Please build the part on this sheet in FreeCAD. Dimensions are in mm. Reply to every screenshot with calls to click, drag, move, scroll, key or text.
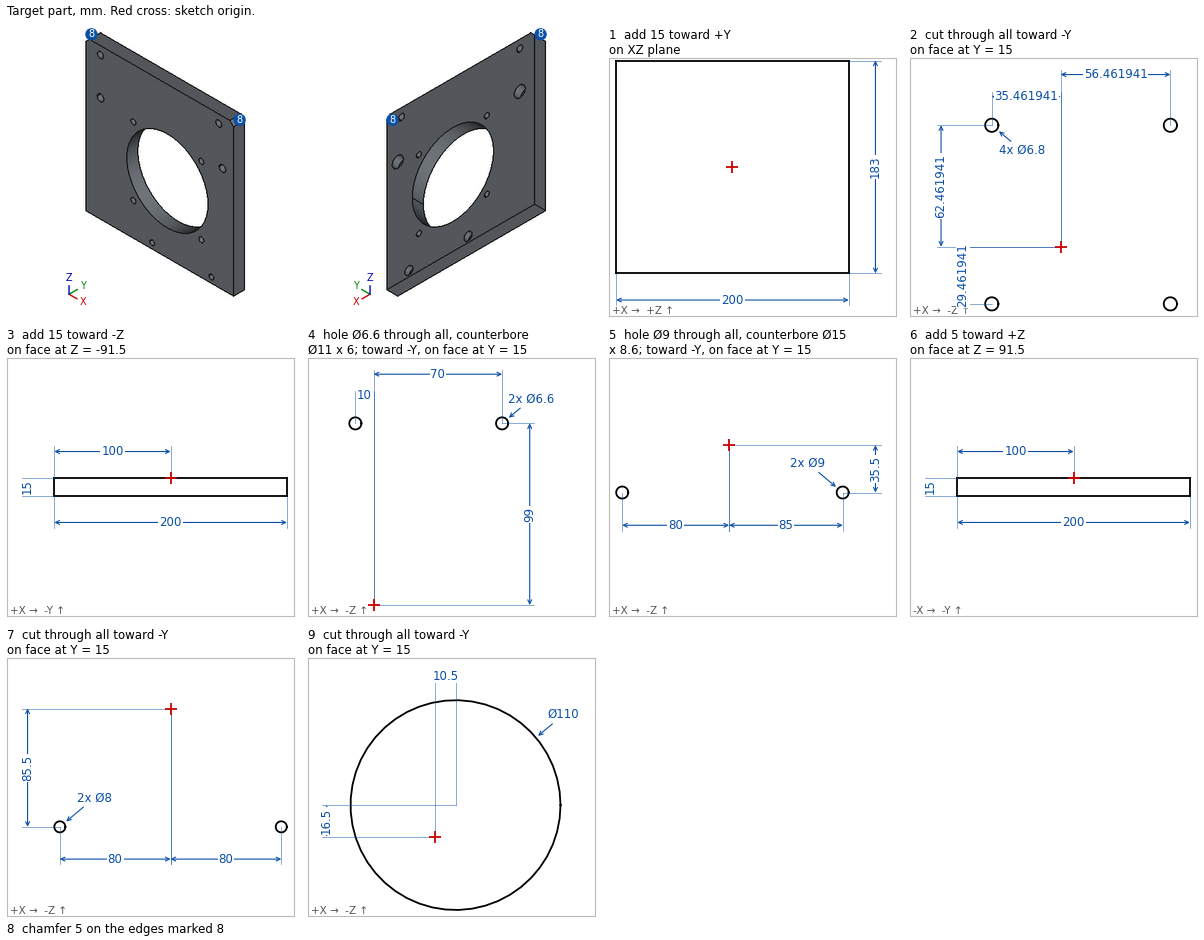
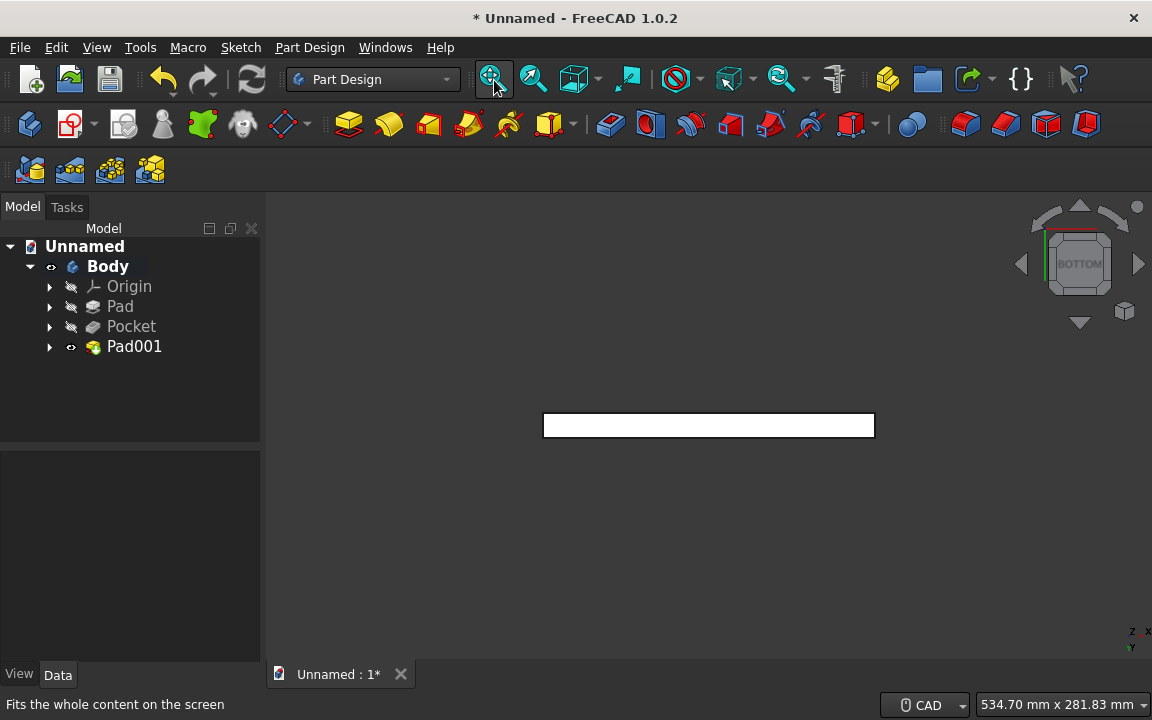
key(4)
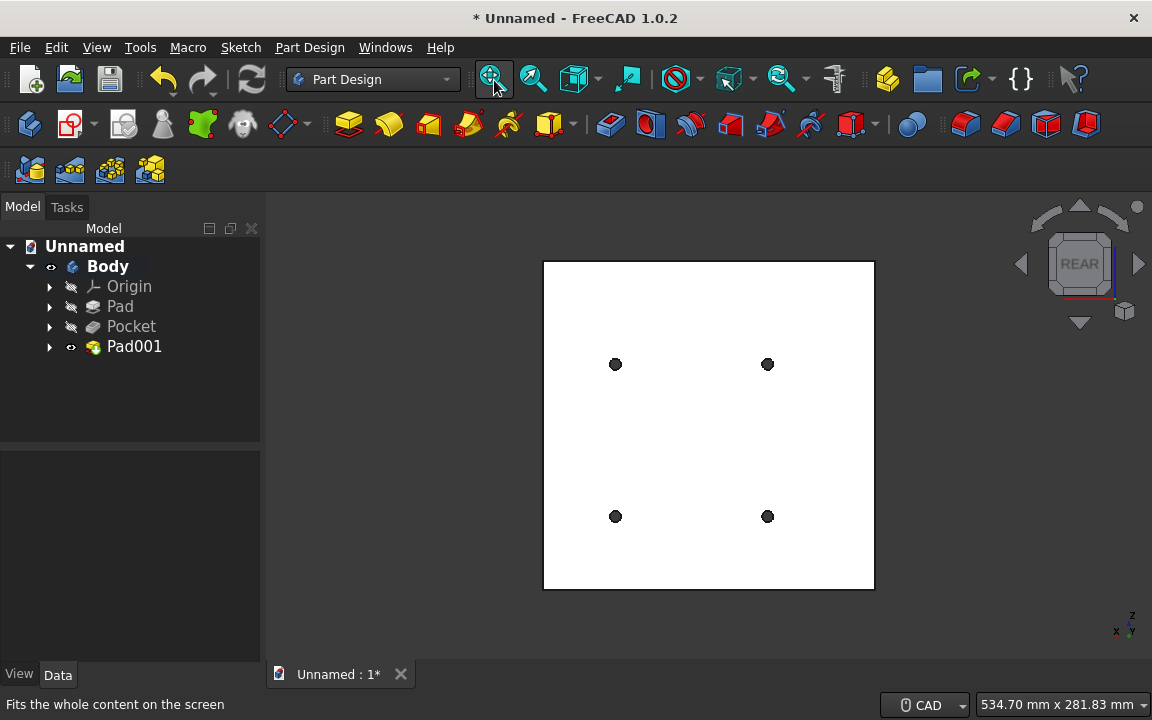
click(709, 424)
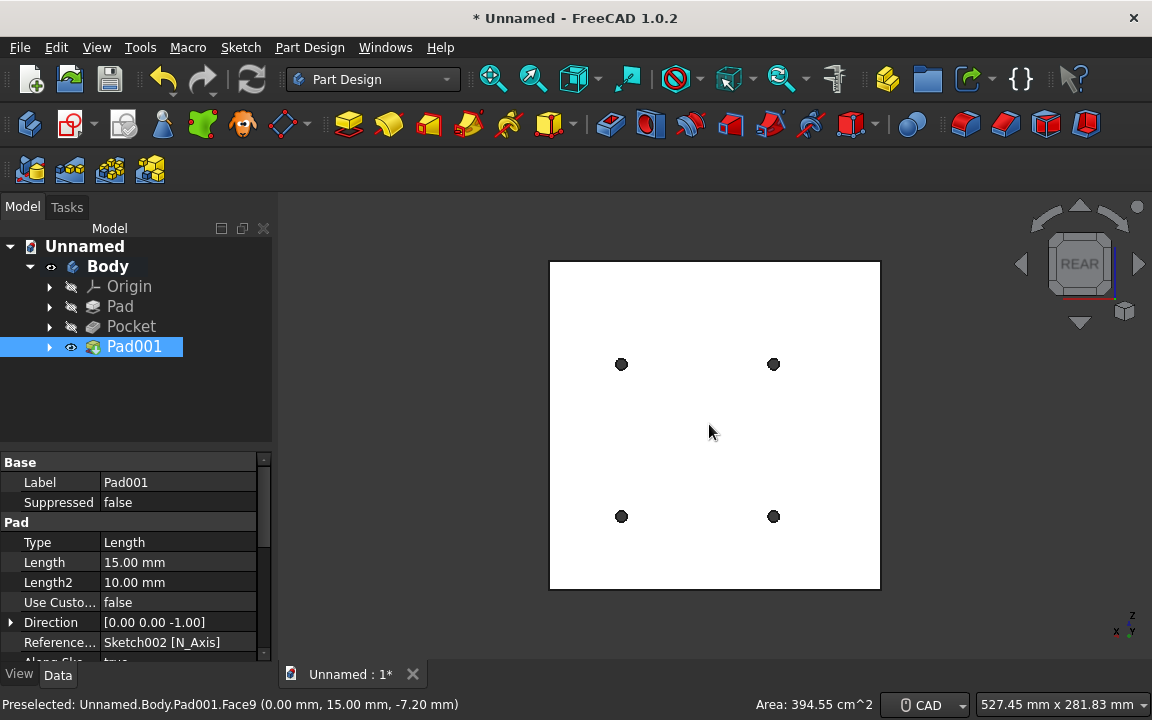
click(70, 124)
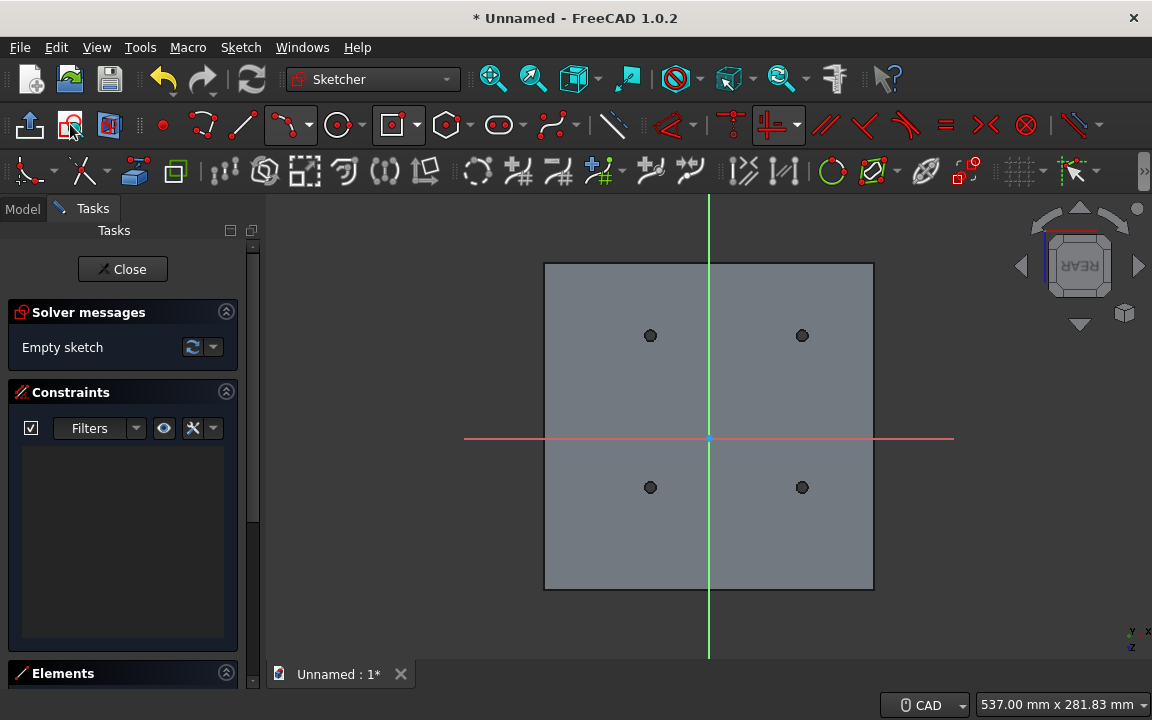
scroll(902, 267, up, 3)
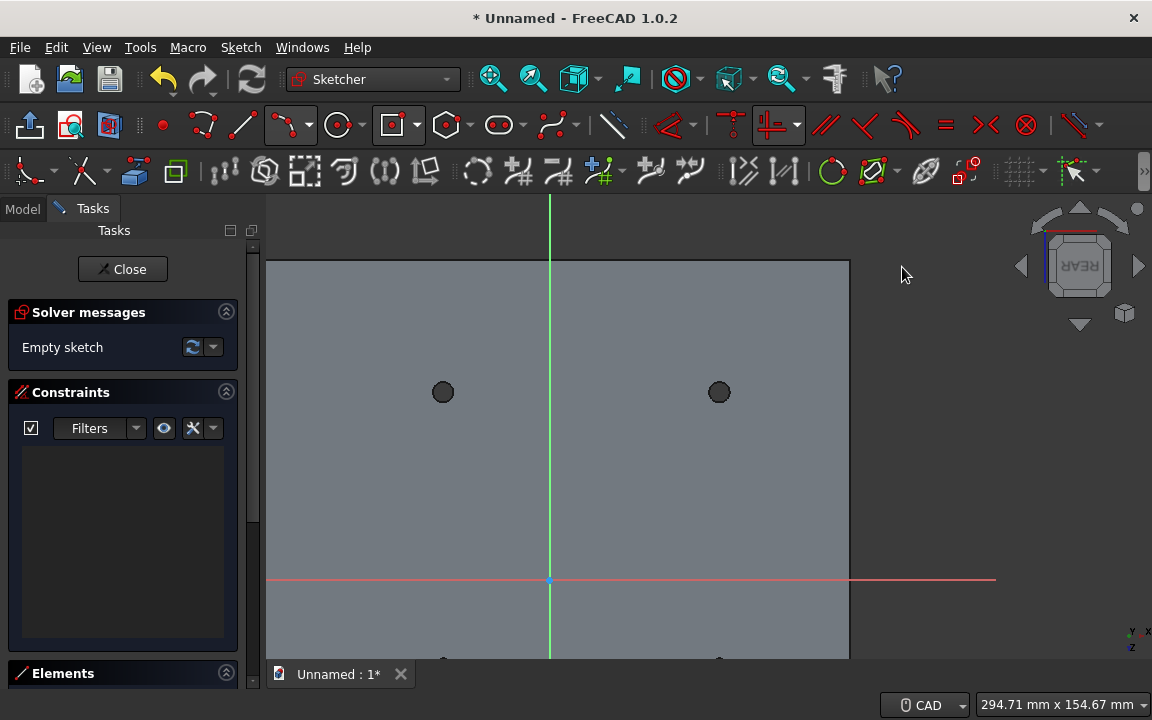
click(338, 126)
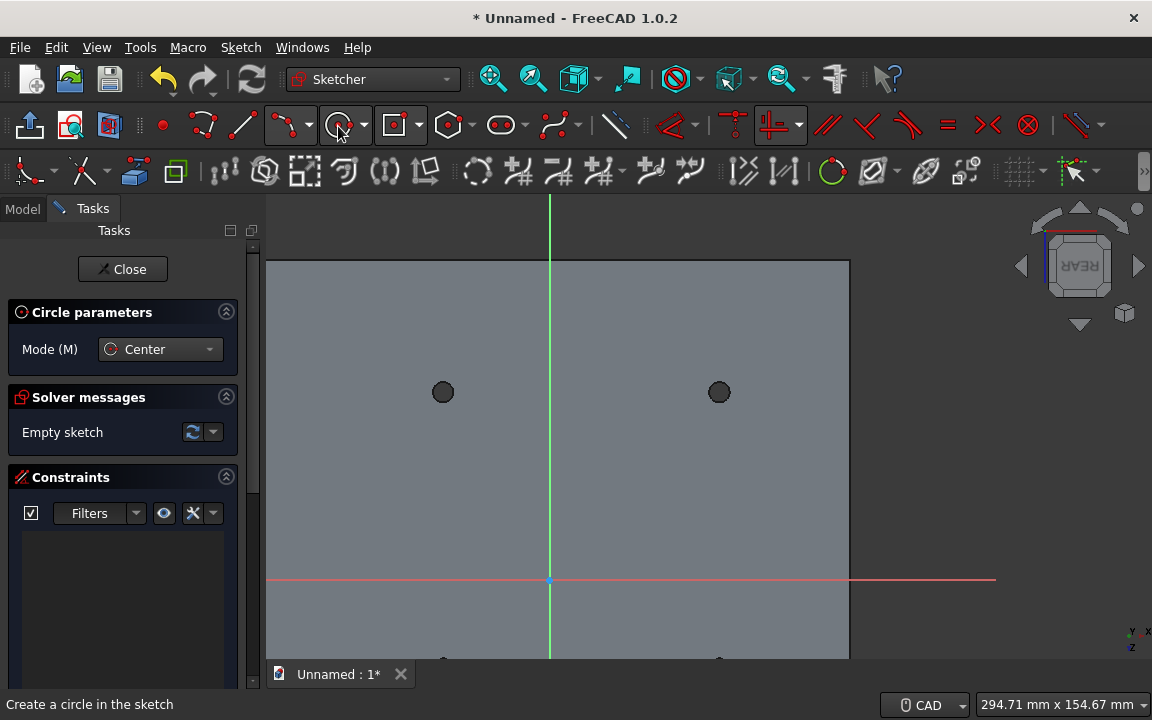
scroll(760, 282, up, 5)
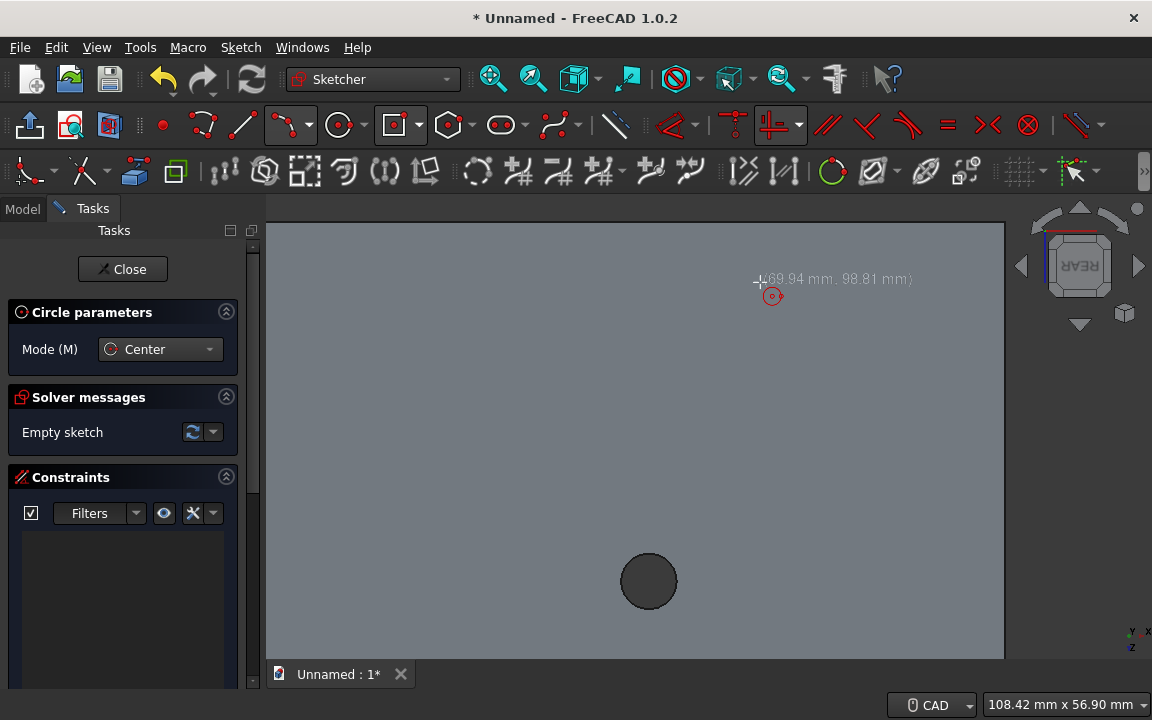
click(760, 283)
click(779, 264)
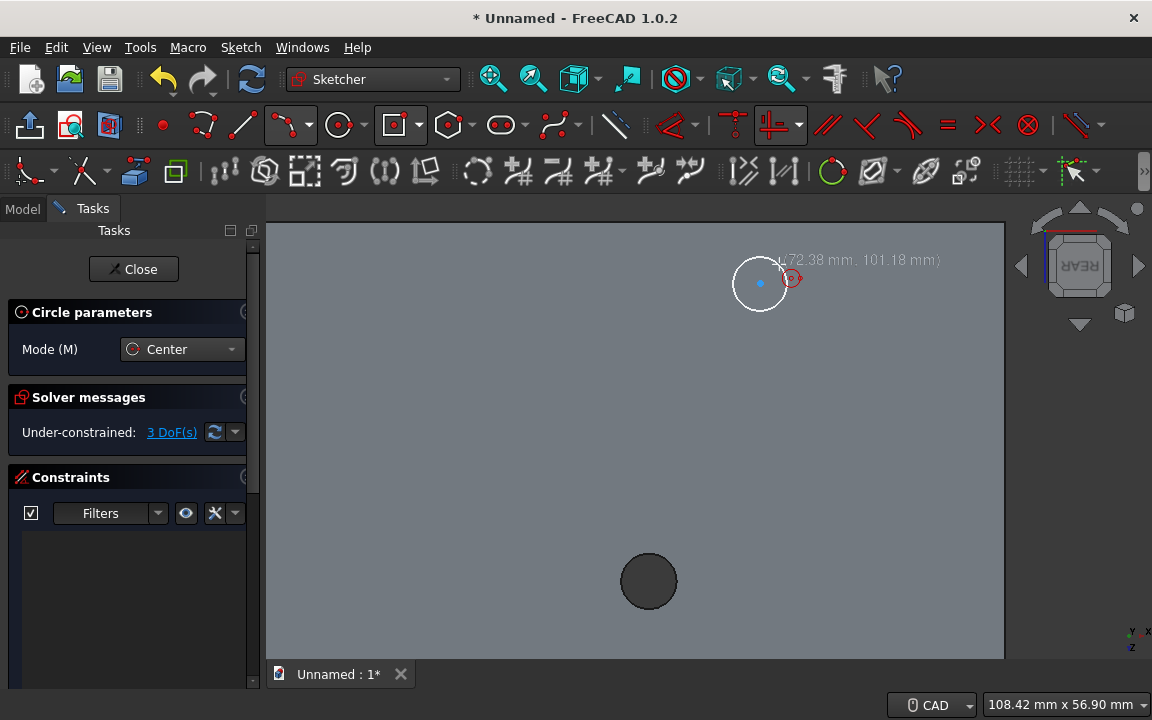
scroll(761, 283, down, 5)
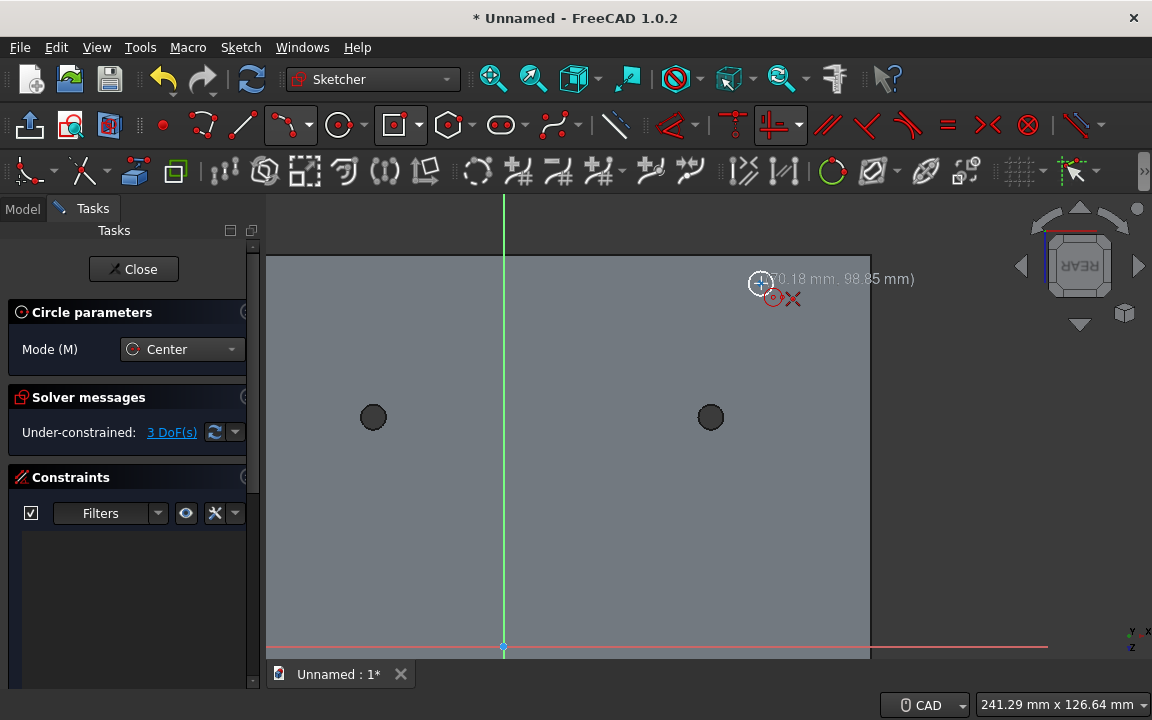
scroll(520, 283, up, 5)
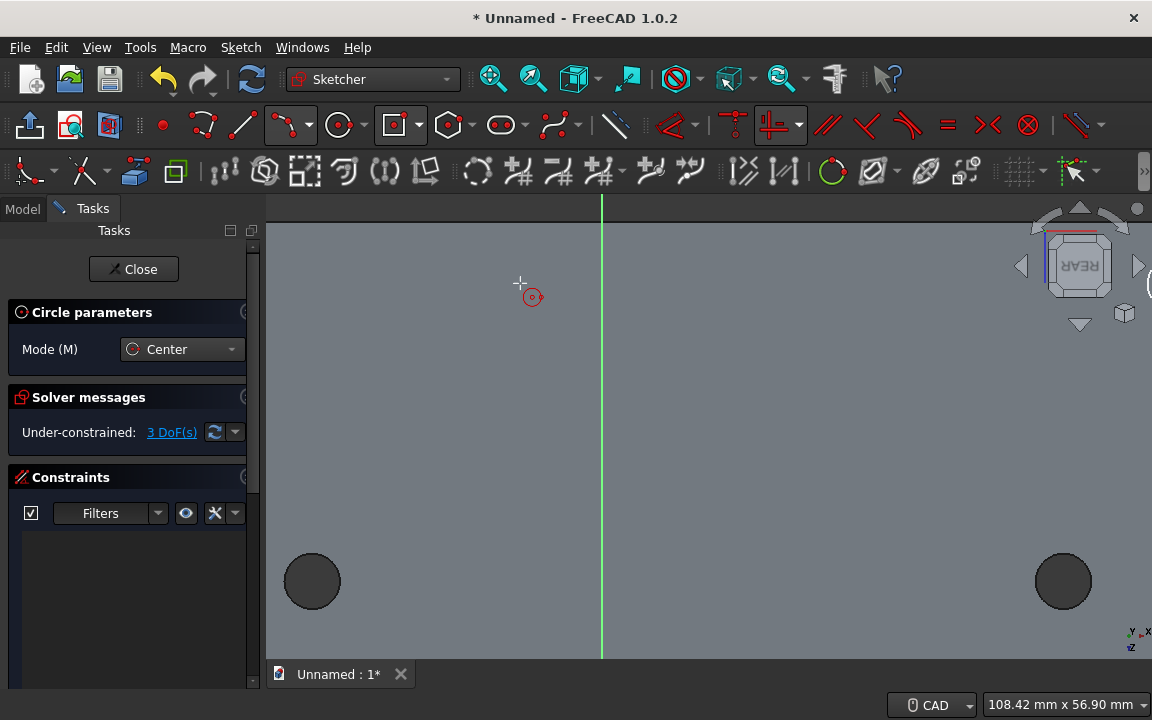
click(520, 283)
click(539, 264)
key(Escape)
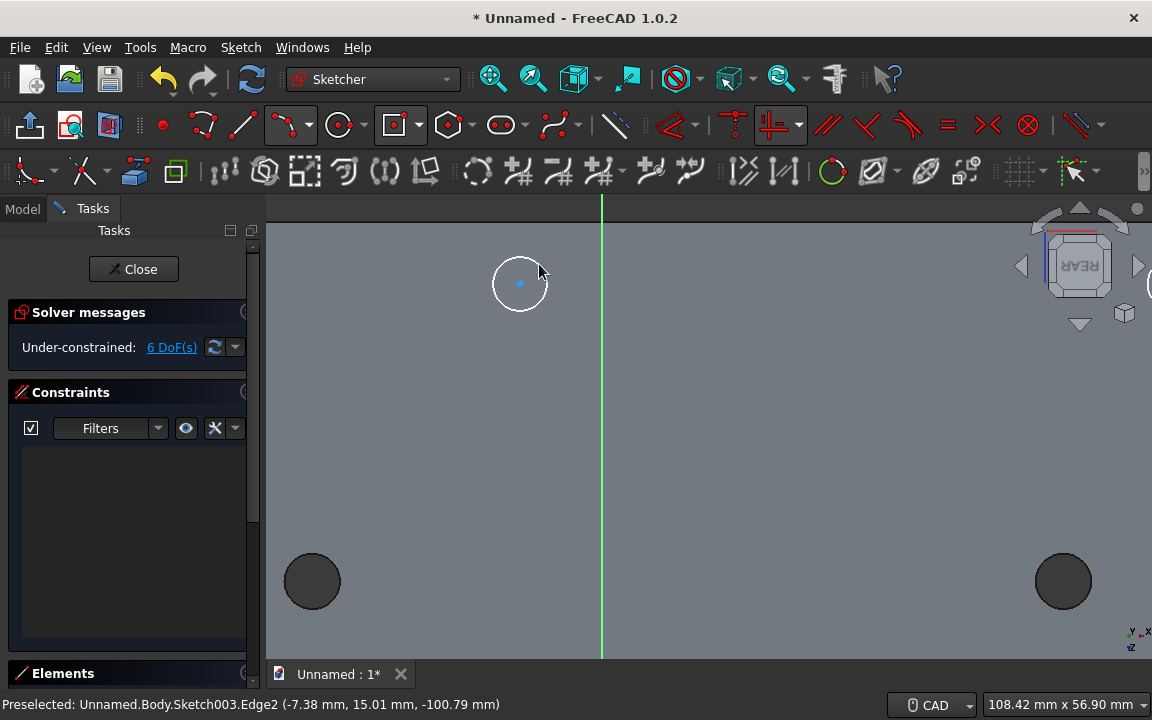
scroll(520, 283, down, 5)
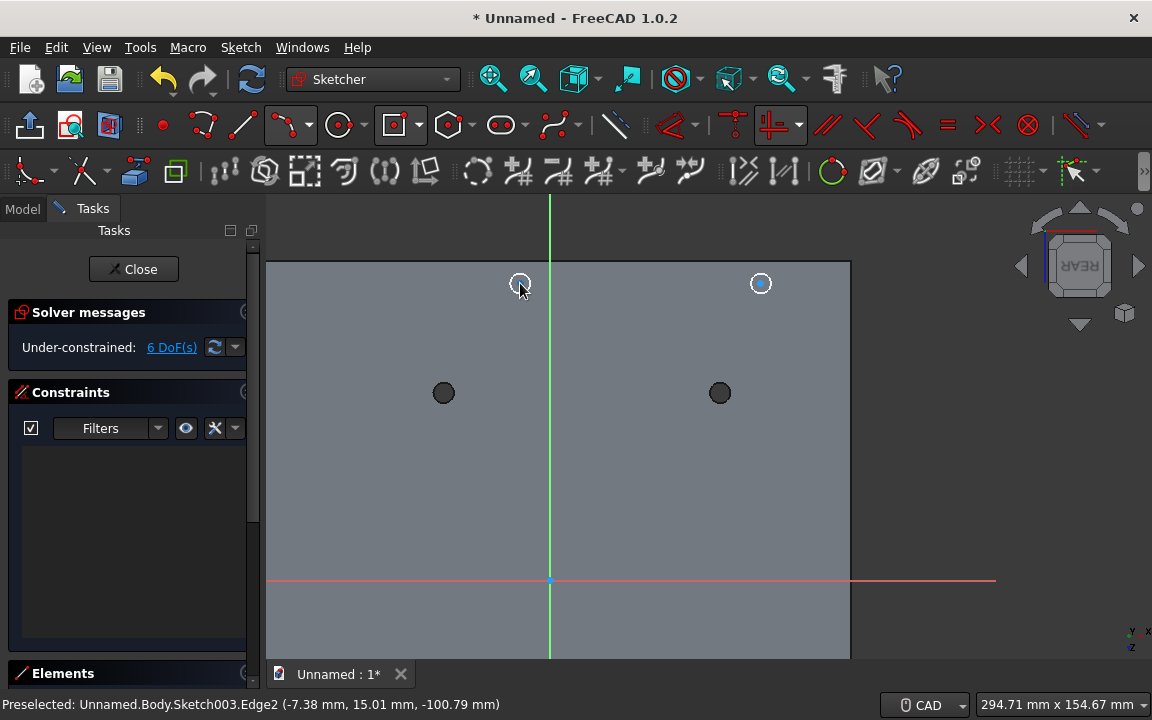
scroll(768, 276, up, 2)